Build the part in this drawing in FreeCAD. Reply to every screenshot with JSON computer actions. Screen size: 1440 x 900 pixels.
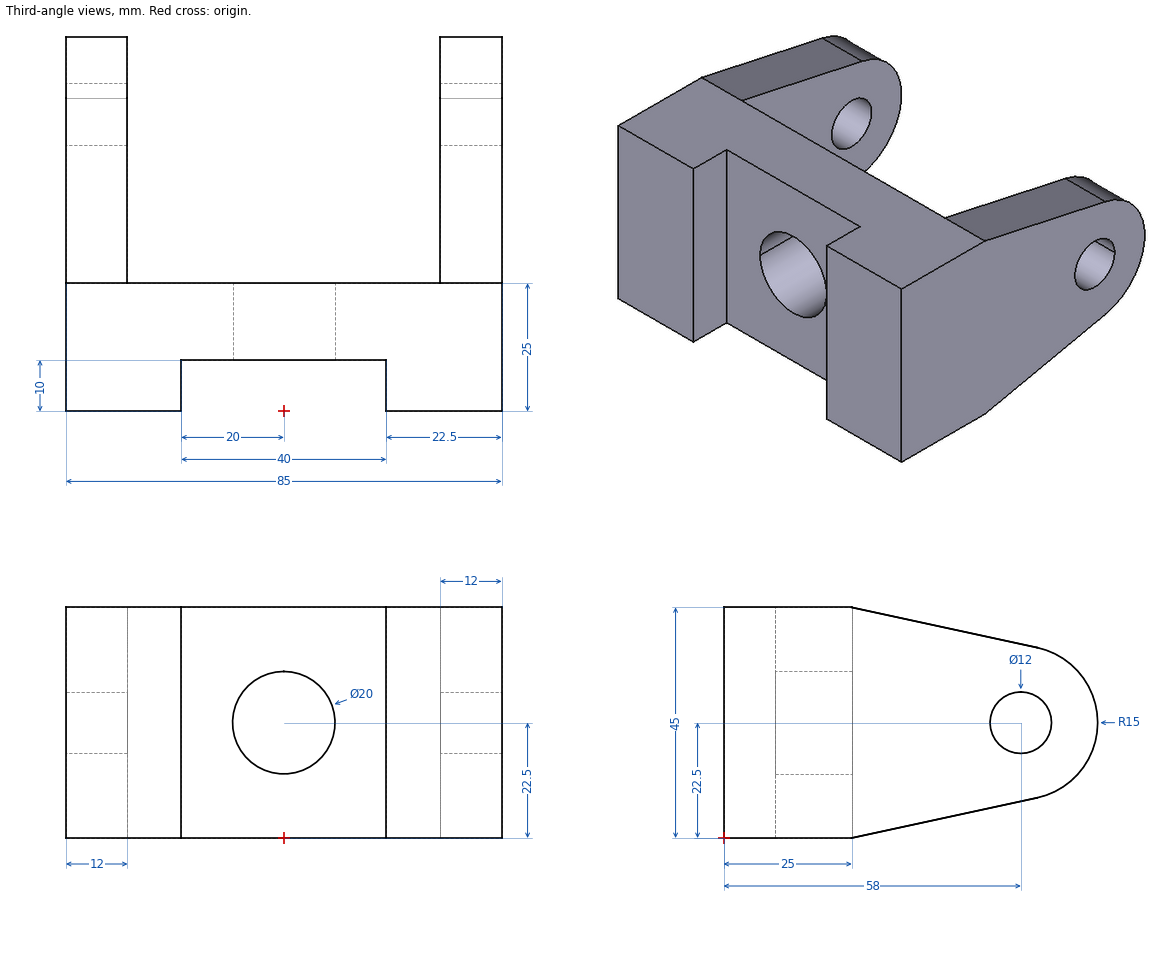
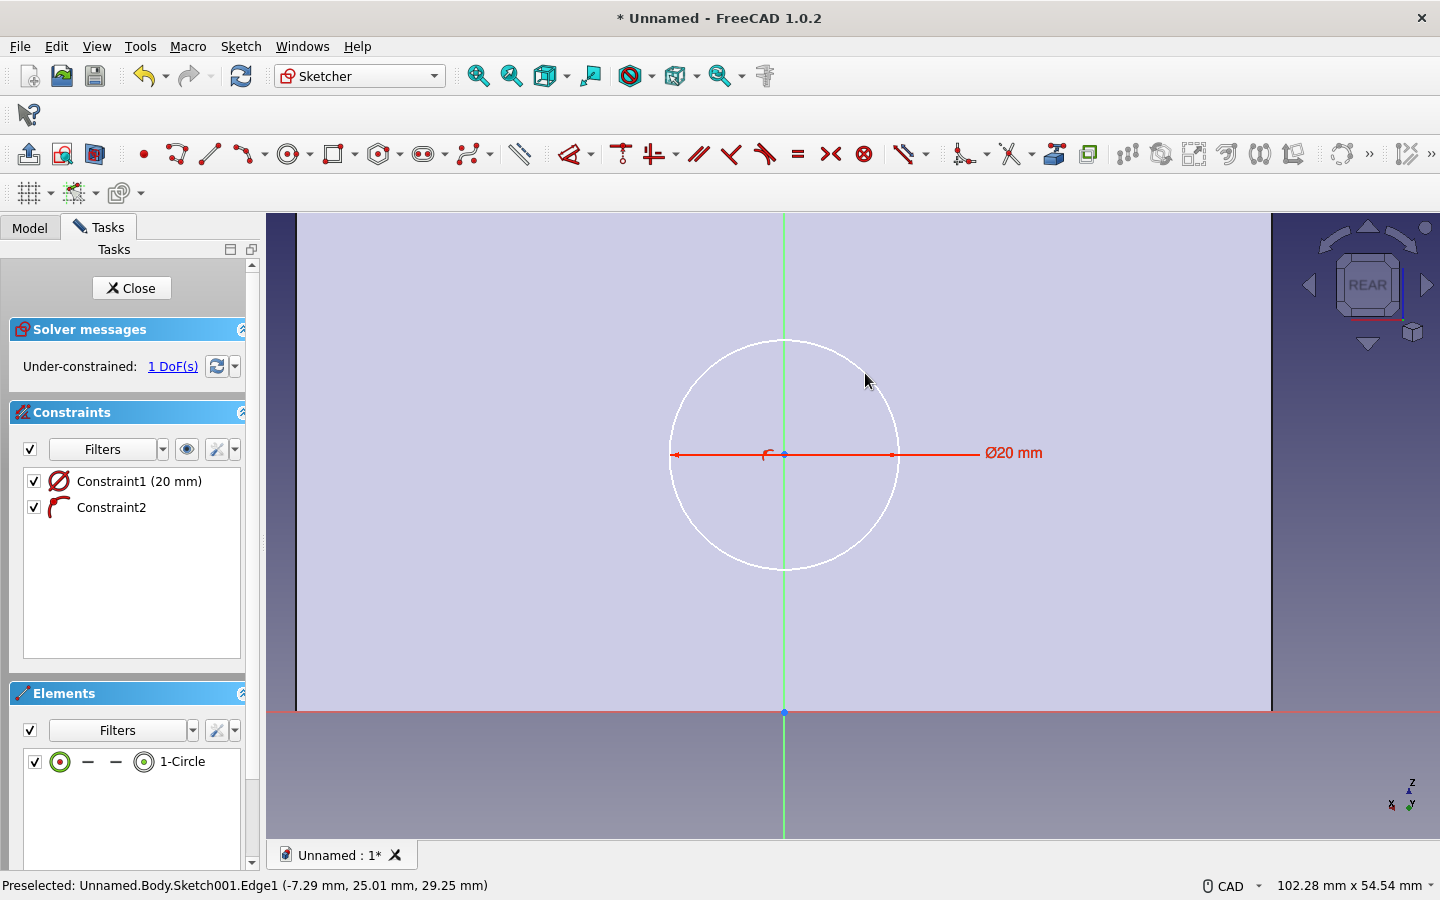
{"action": "left_click", "coordinate": [568, 154]}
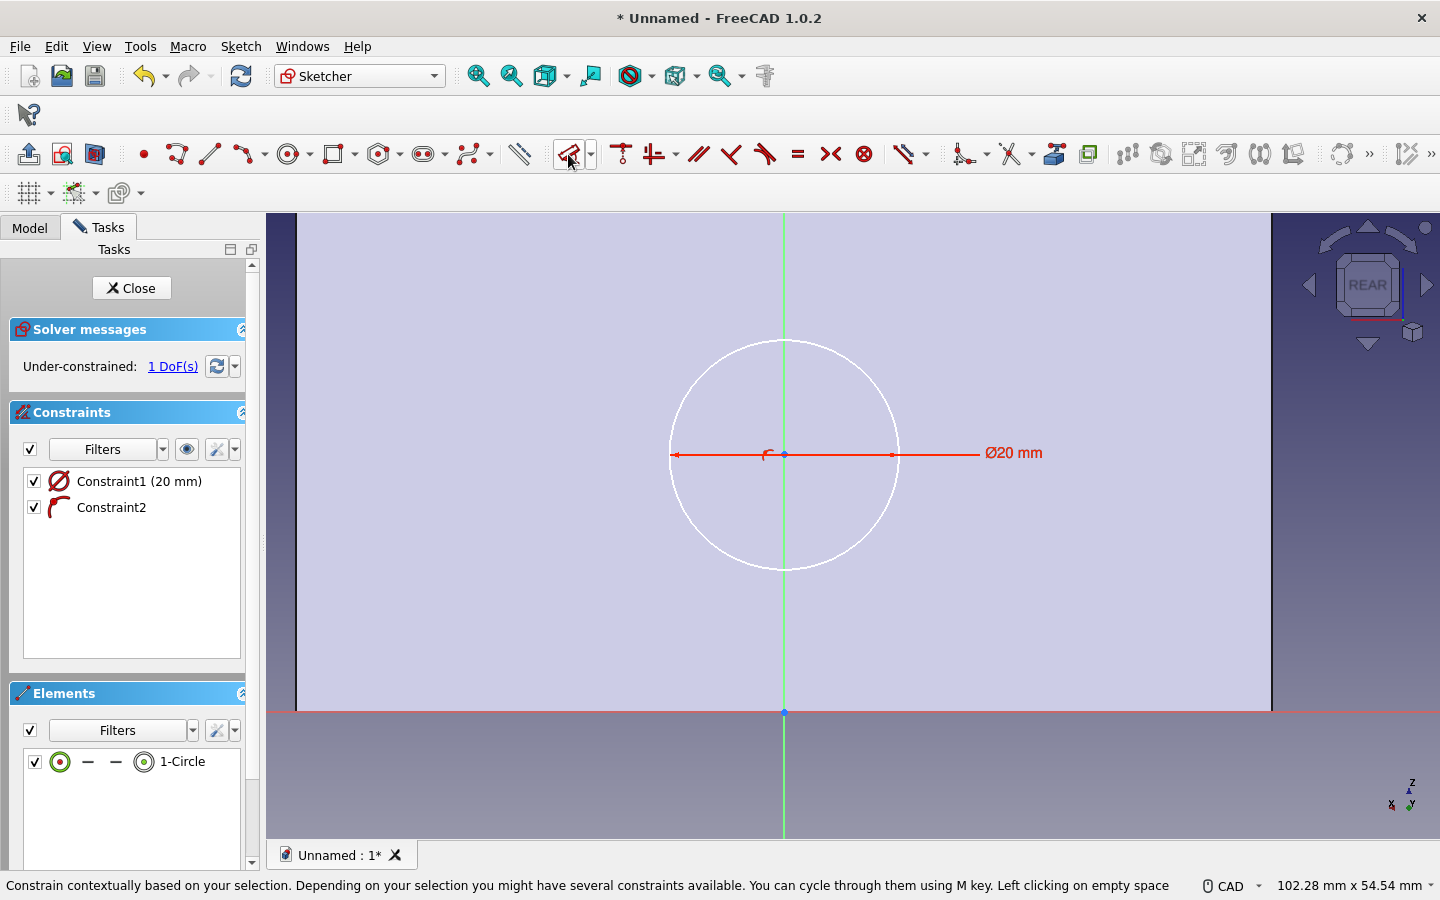
{"action": "left_click", "coordinate": [784, 455]}
{"action": "left_click", "coordinate": [818, 584]}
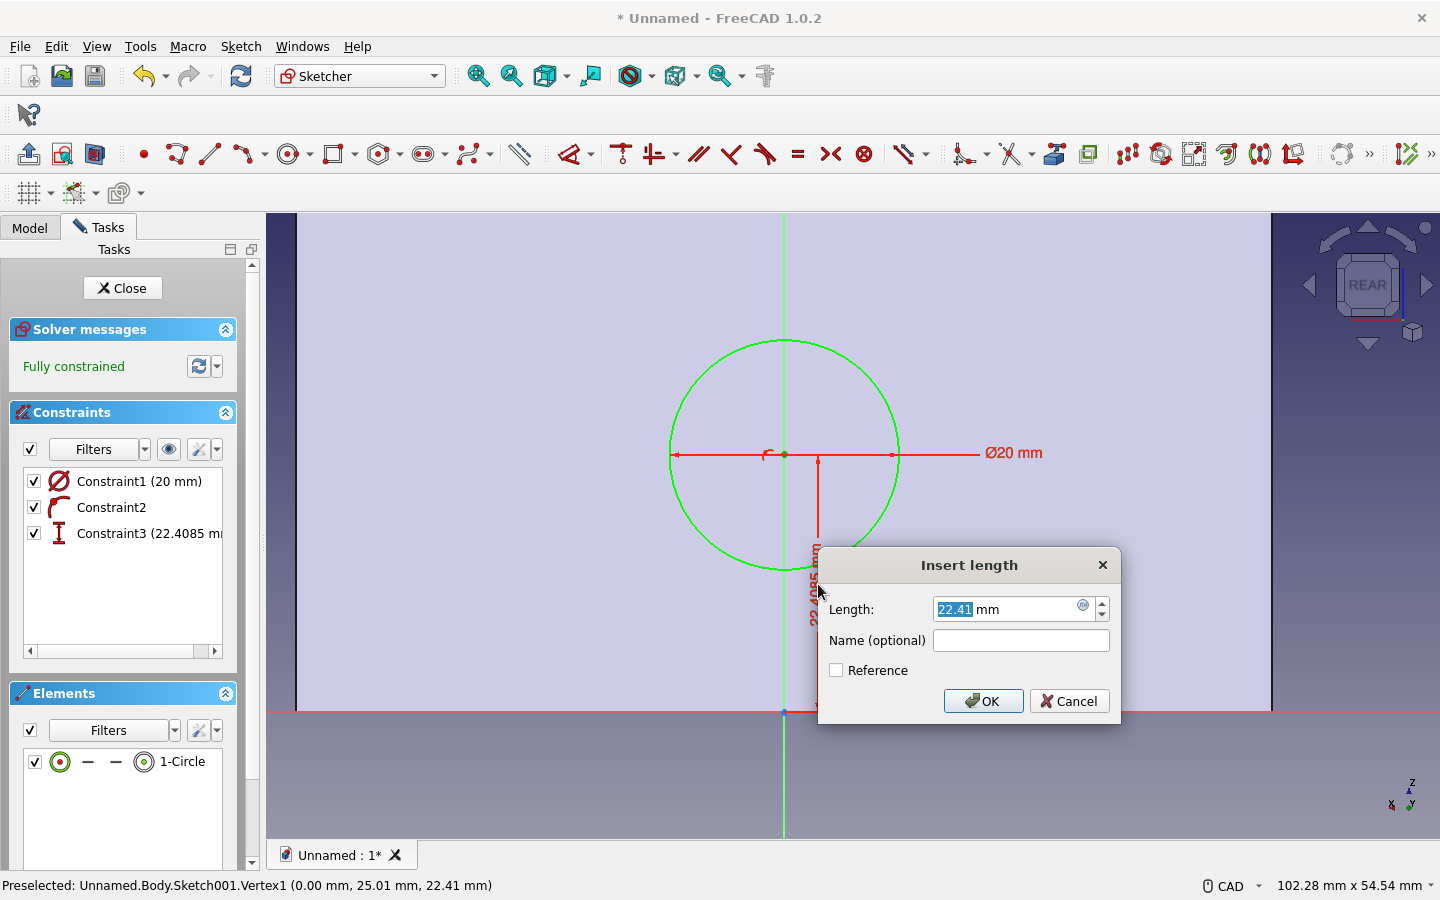
{"action": "type", "text": "22.5"}
{"action": "key", "text": "Return"}
{"action": "key", "text": "Escape"}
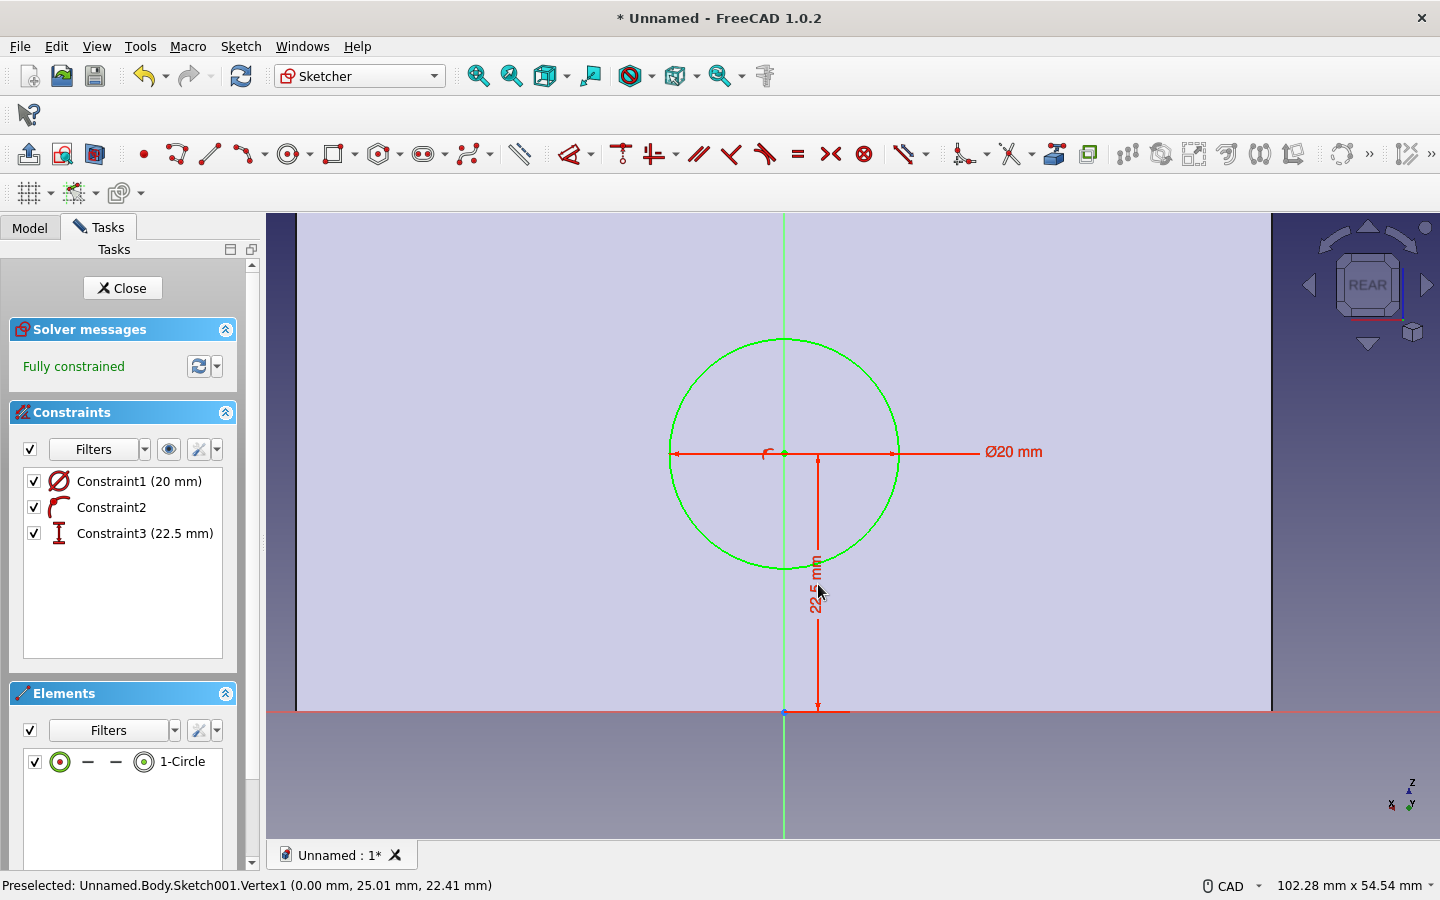
{"action": "left_click", "coordinate": [123, 288]}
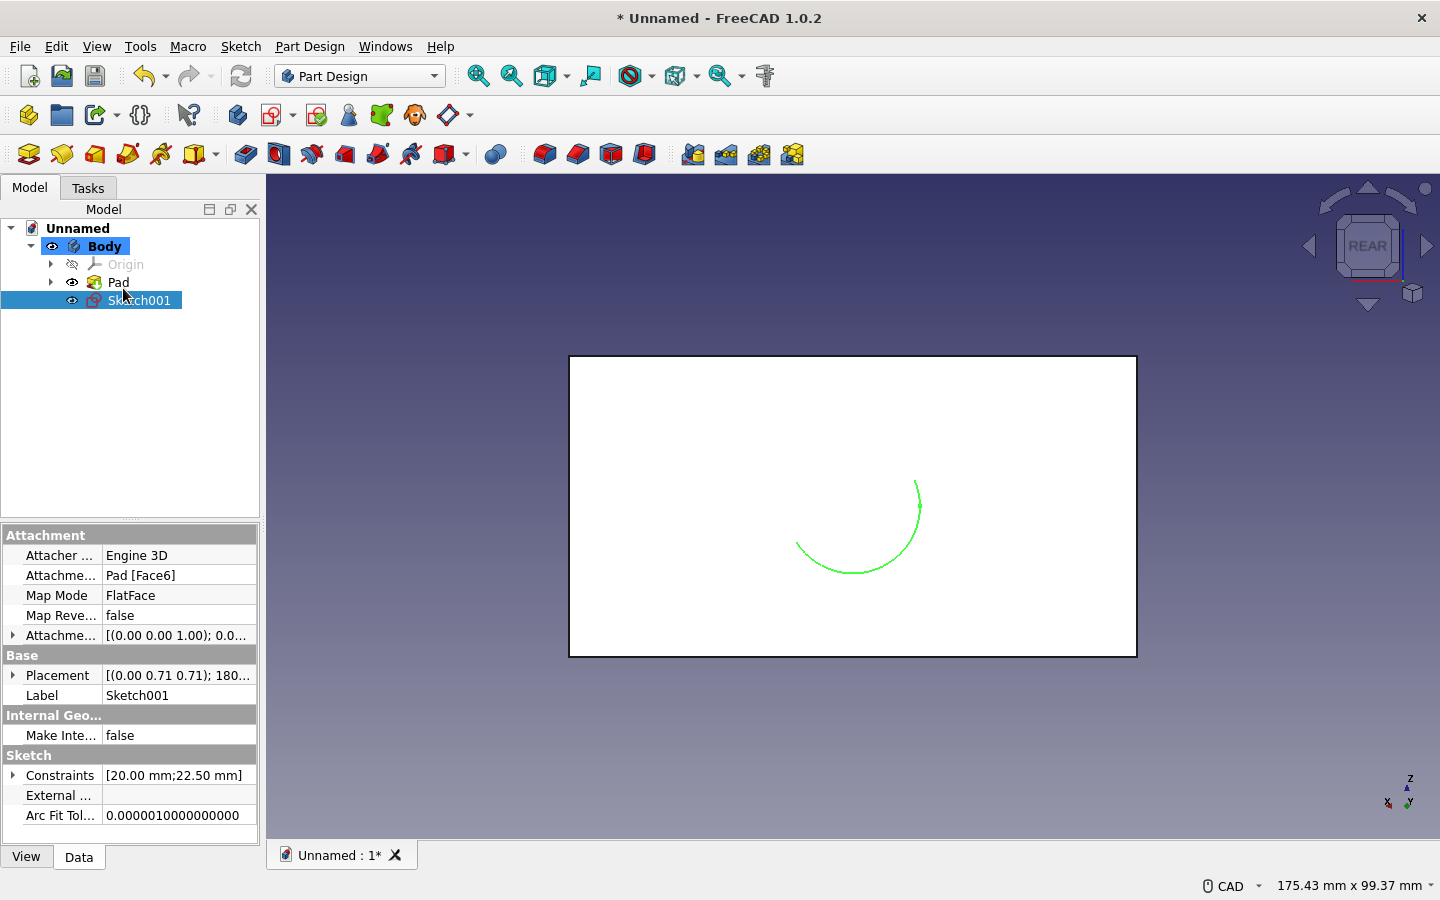
{"action": "left_click", "coordinate": [246, 154]}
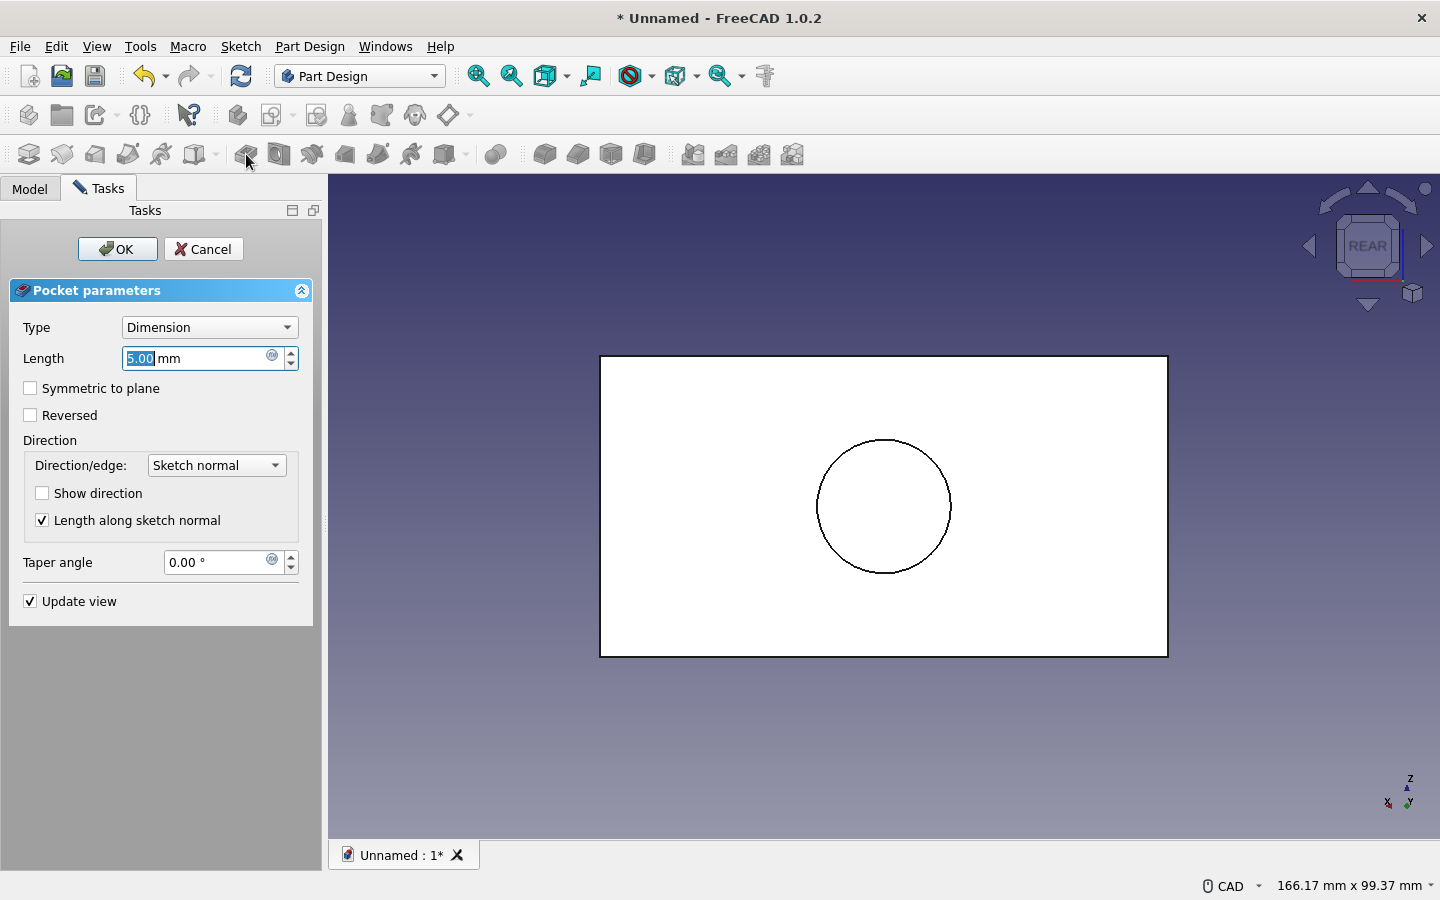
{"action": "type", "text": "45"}
{"action": "key", "text": "Tab"}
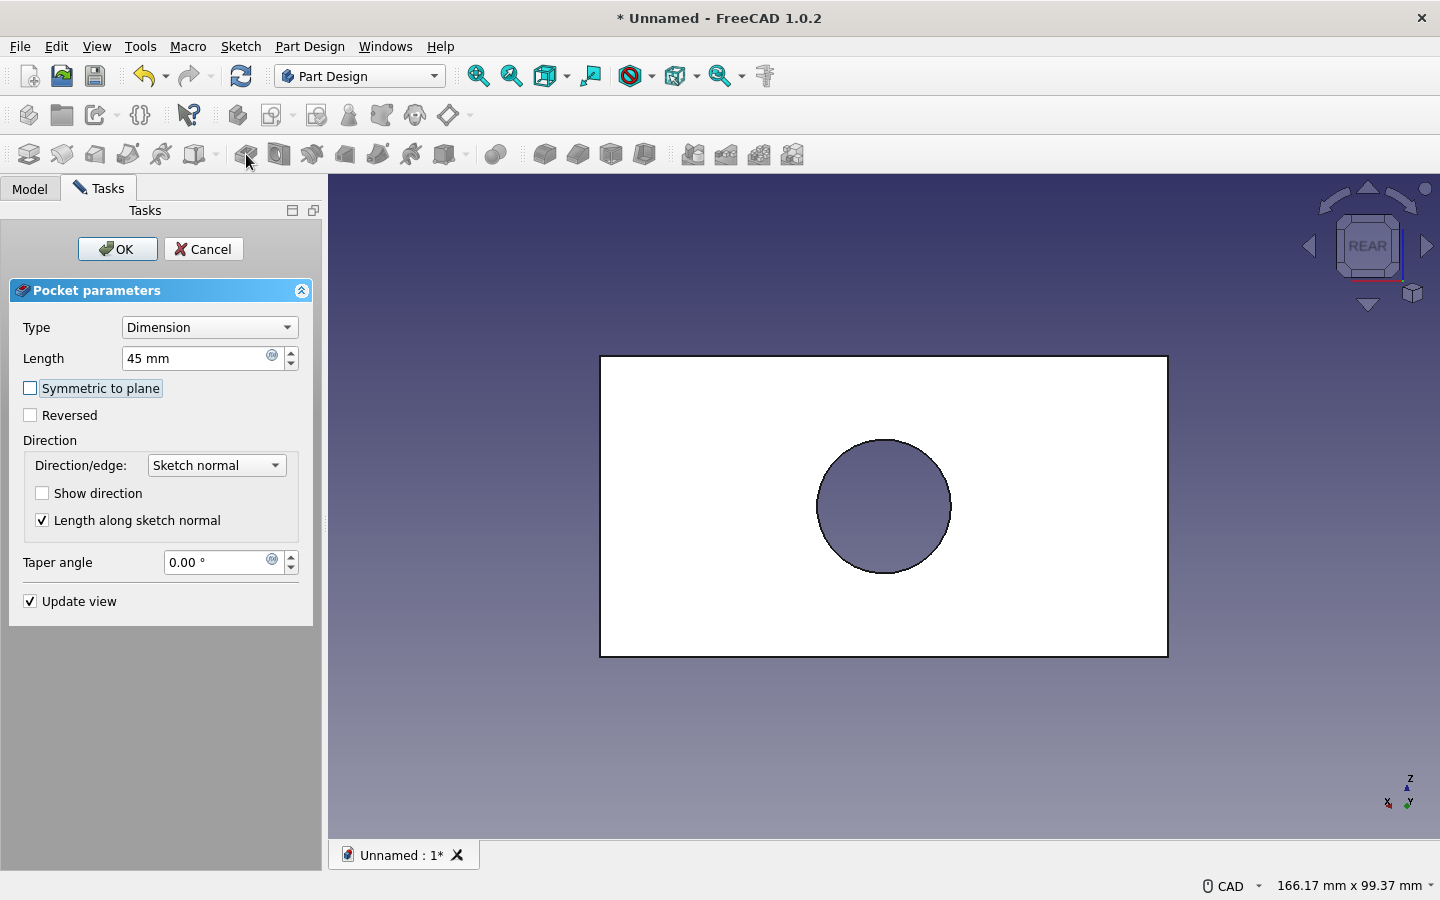
{"action": "left_click", "coordinate": [118, 249]}